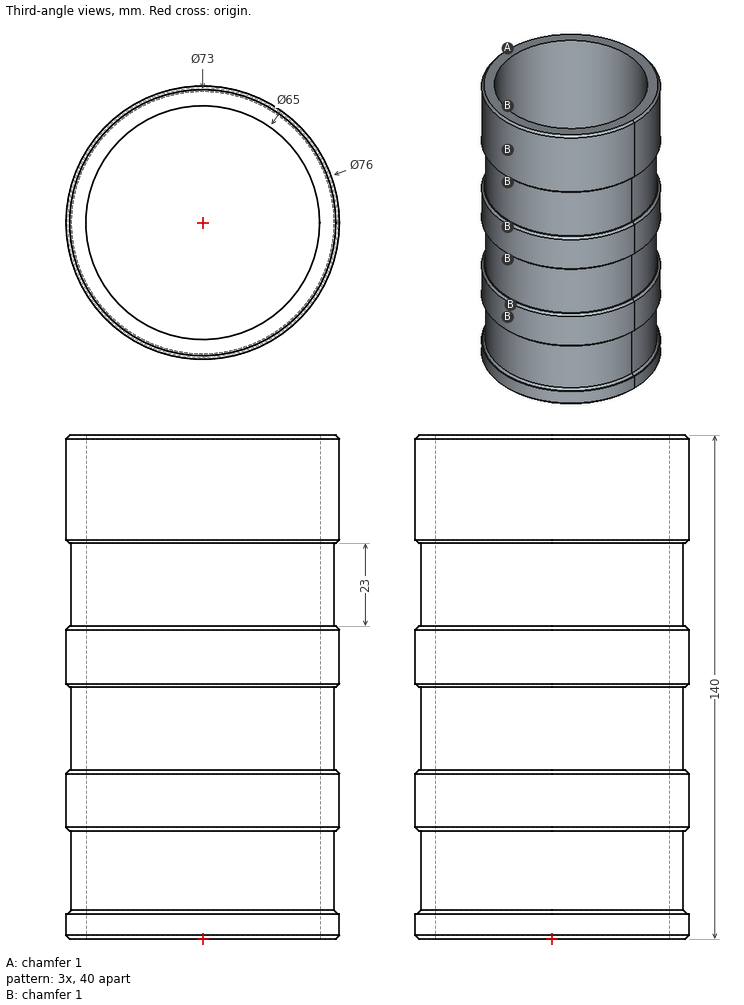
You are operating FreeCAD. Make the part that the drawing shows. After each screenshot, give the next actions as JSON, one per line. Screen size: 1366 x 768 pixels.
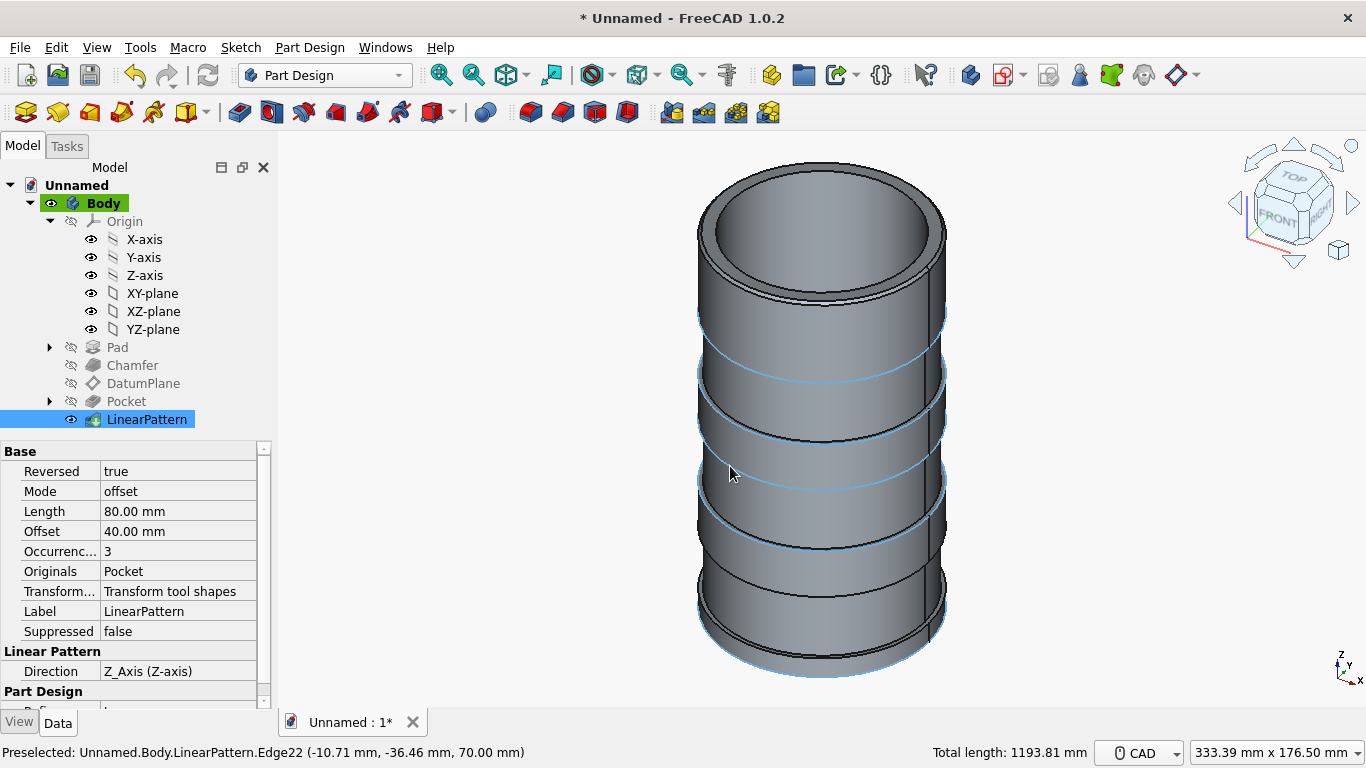
{"action": "left_click", "coordinate": [730, 573], "text": "ctrl"}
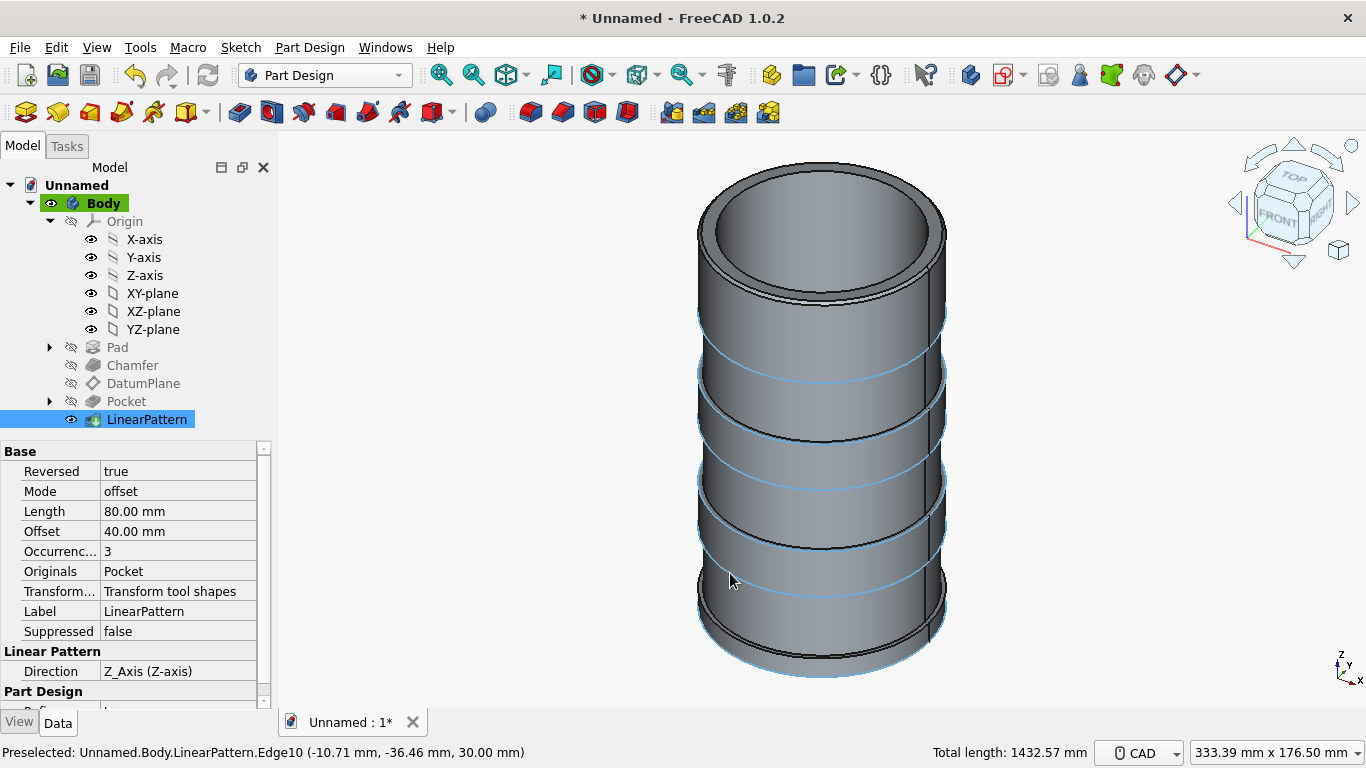
{"action": "key", "text": "0"}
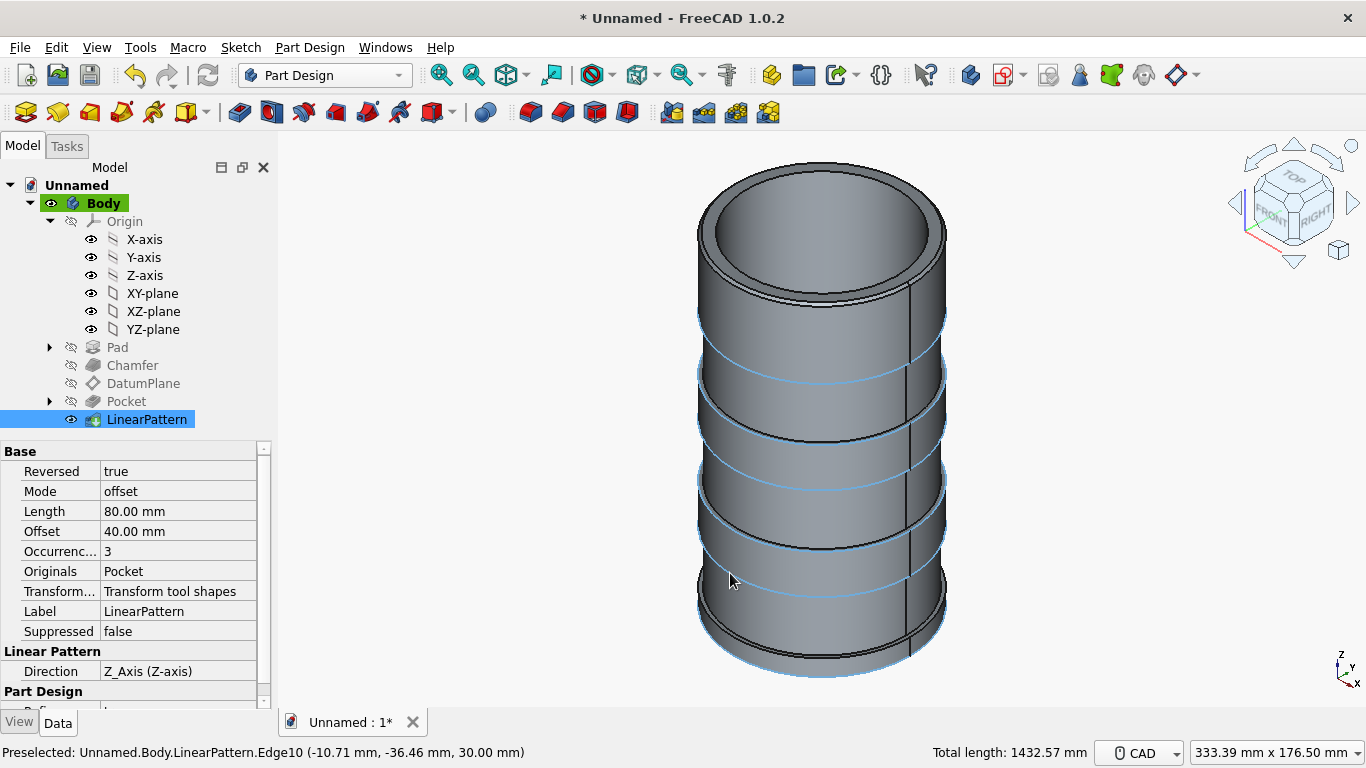
{"action": "left_click", "coordinate": [442, 76]}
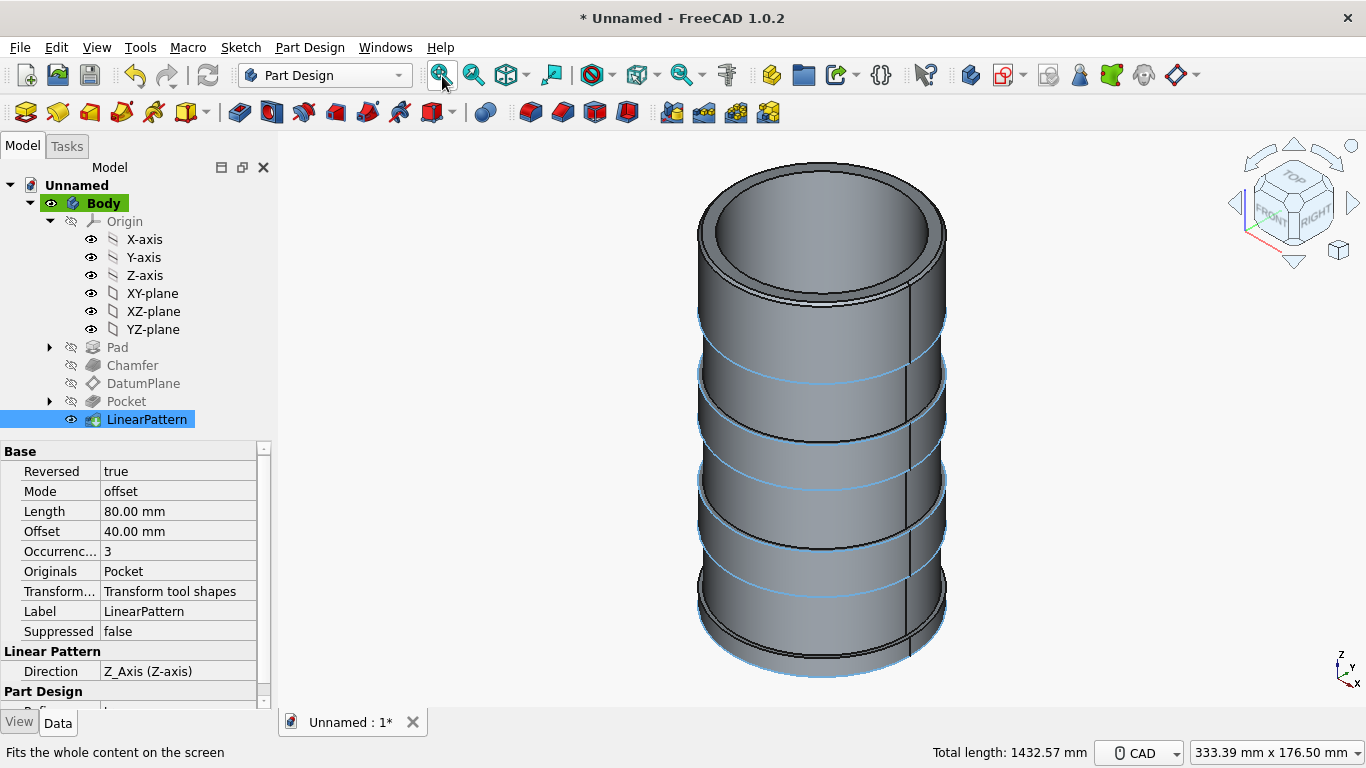
{"action": "key", "text": "2"}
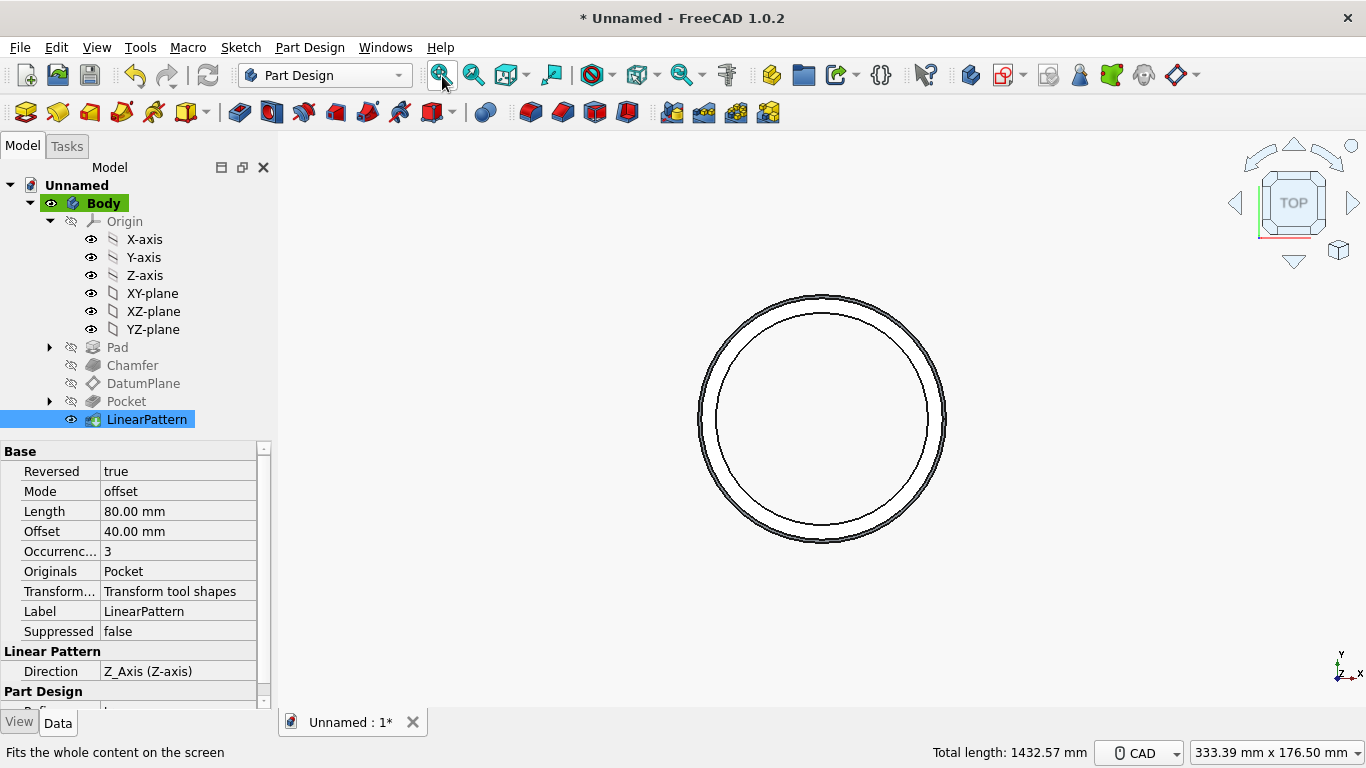
{"action": "key", "text": "v f"}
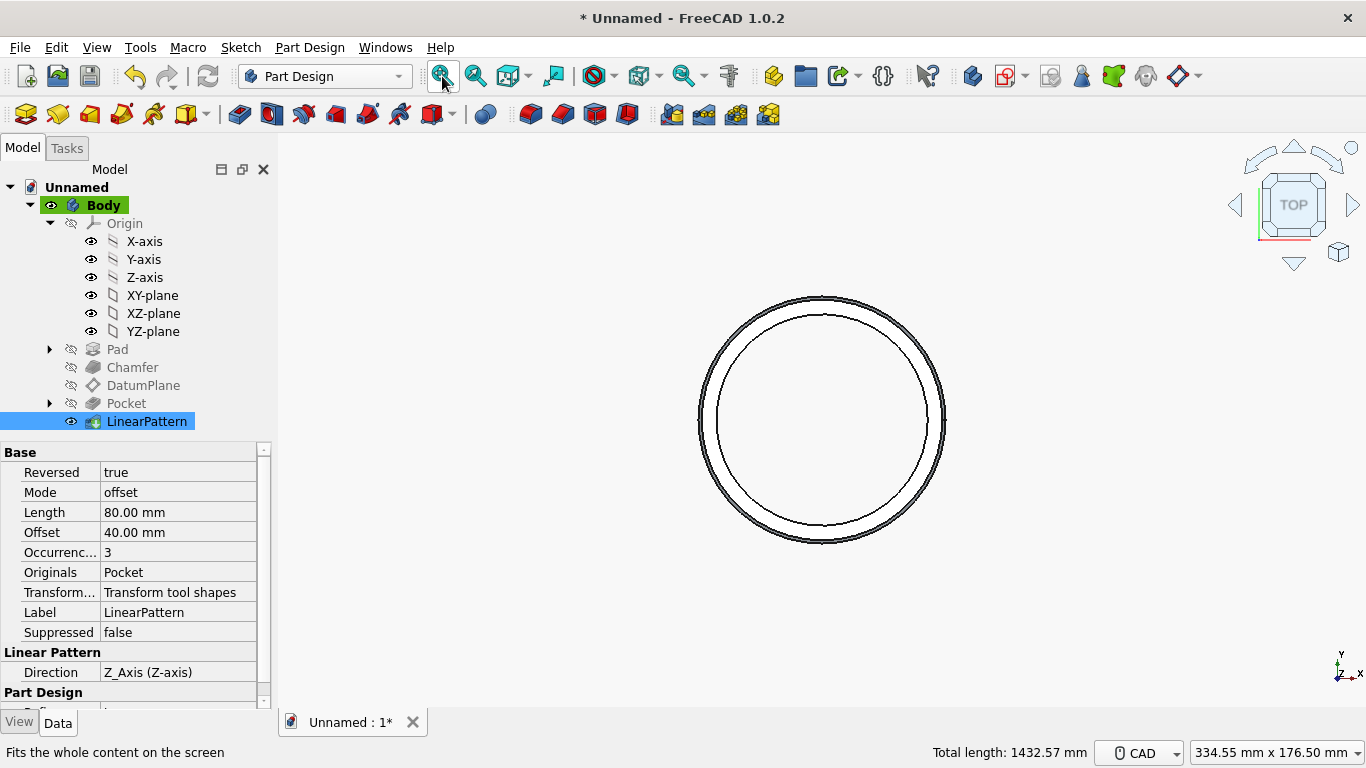
{"action": "key", "text": "1"}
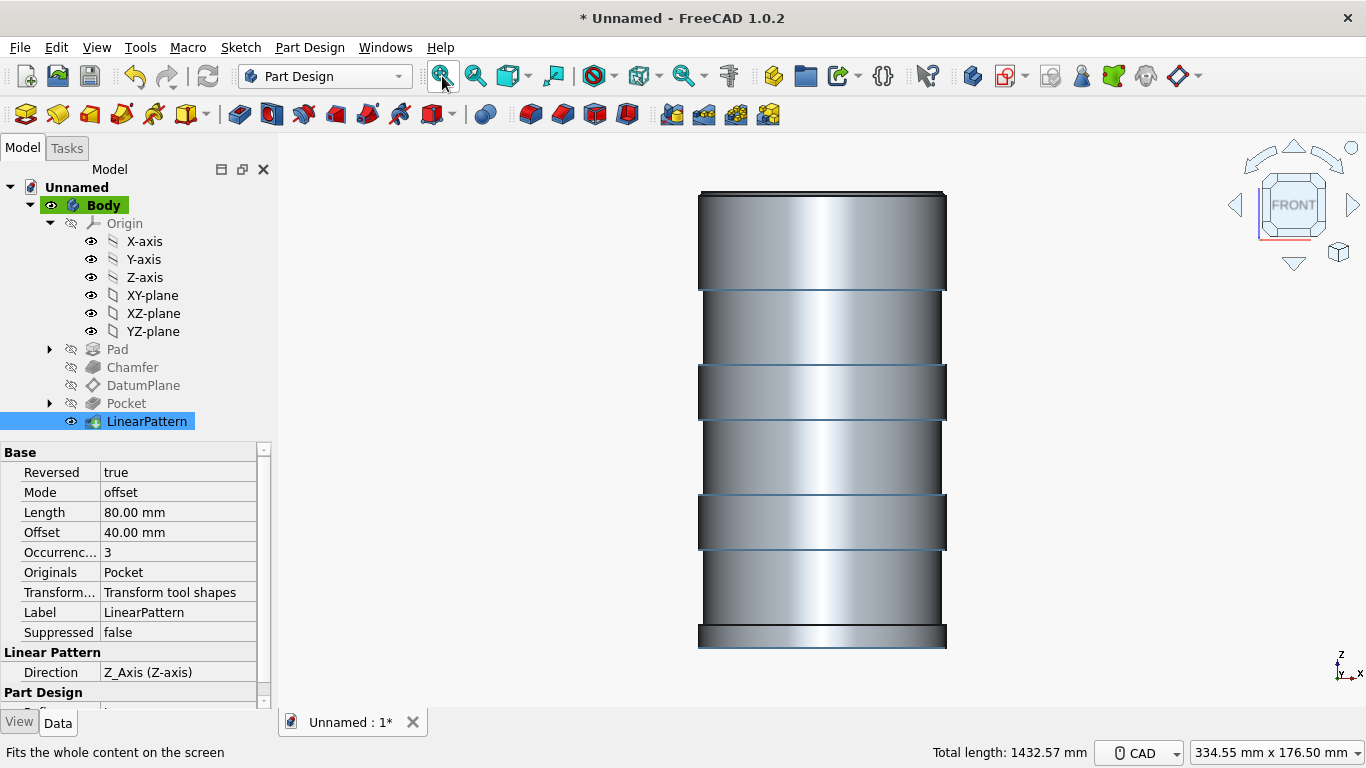
{"action": "key", "text": "3"}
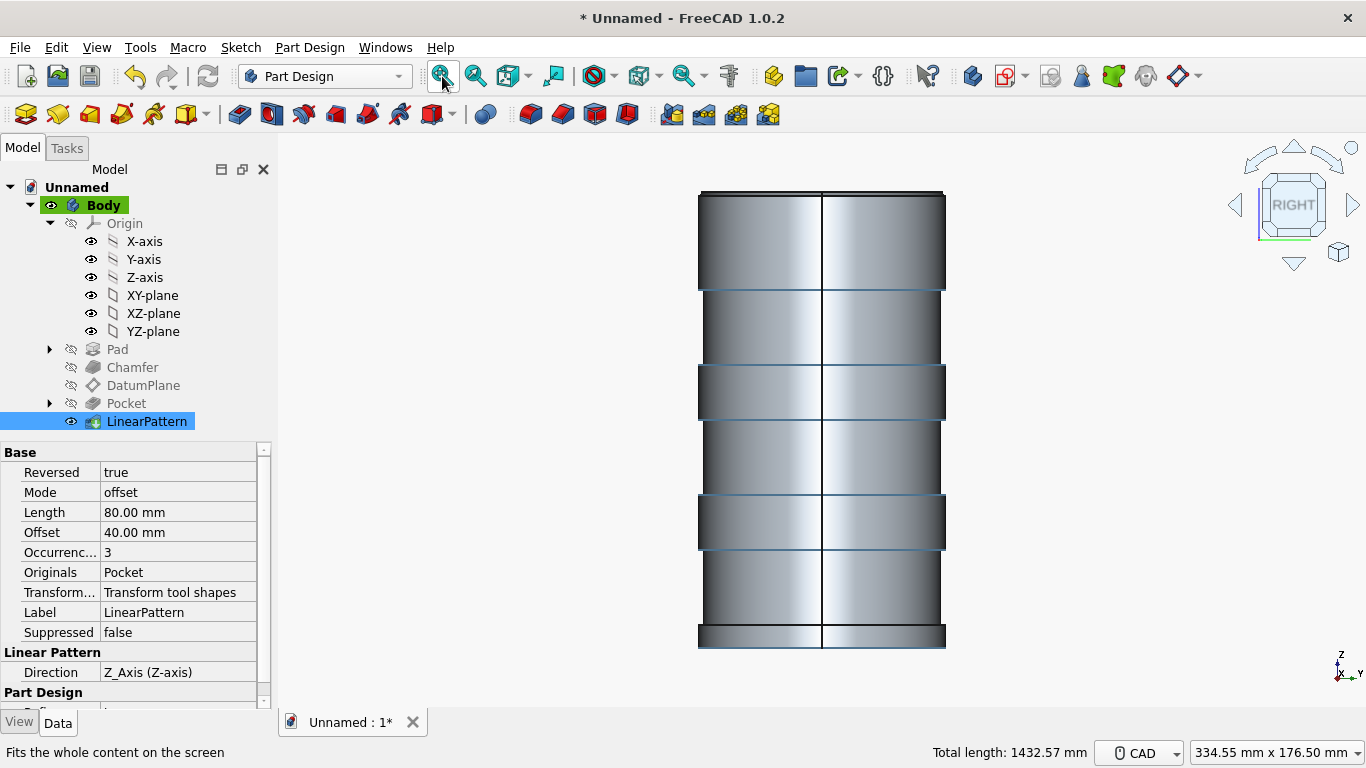
{"action": "key", "text": "5"}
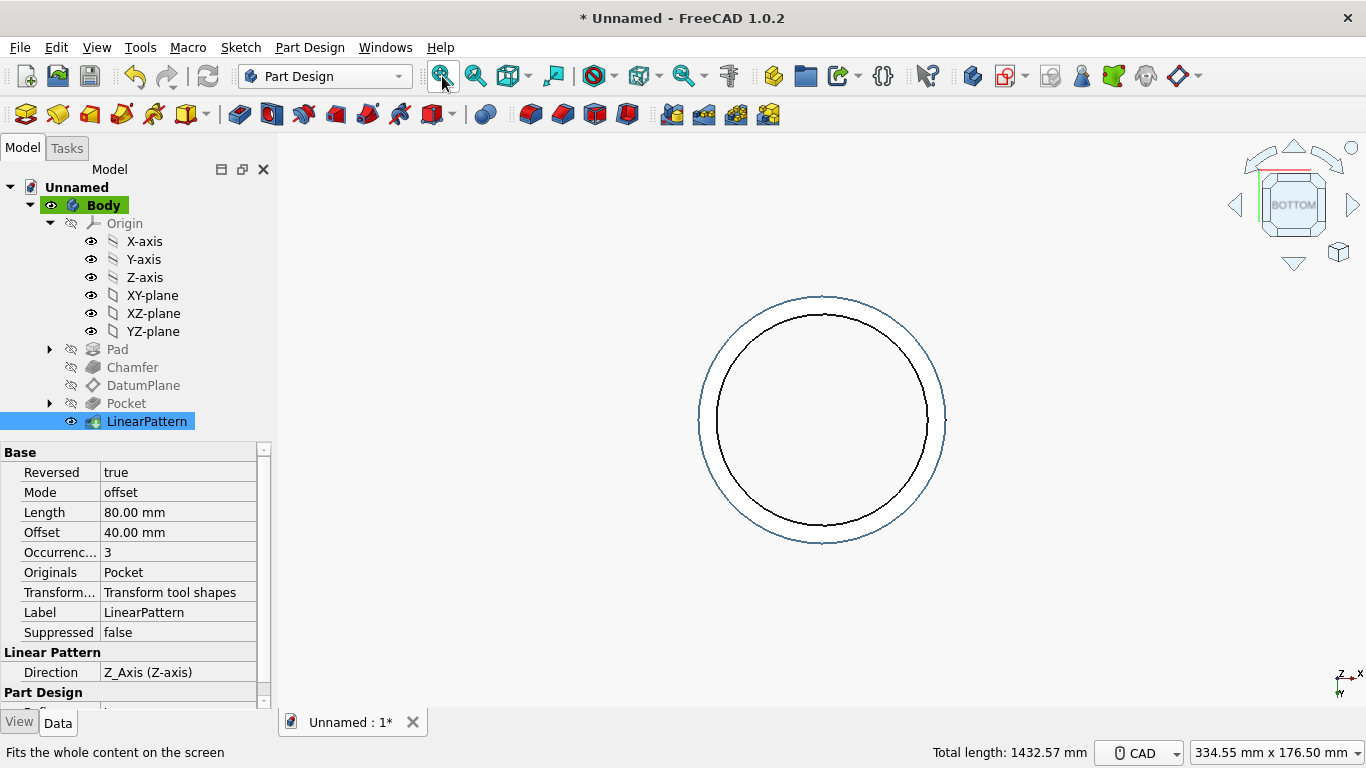
{"action": "key", "text": "v f"}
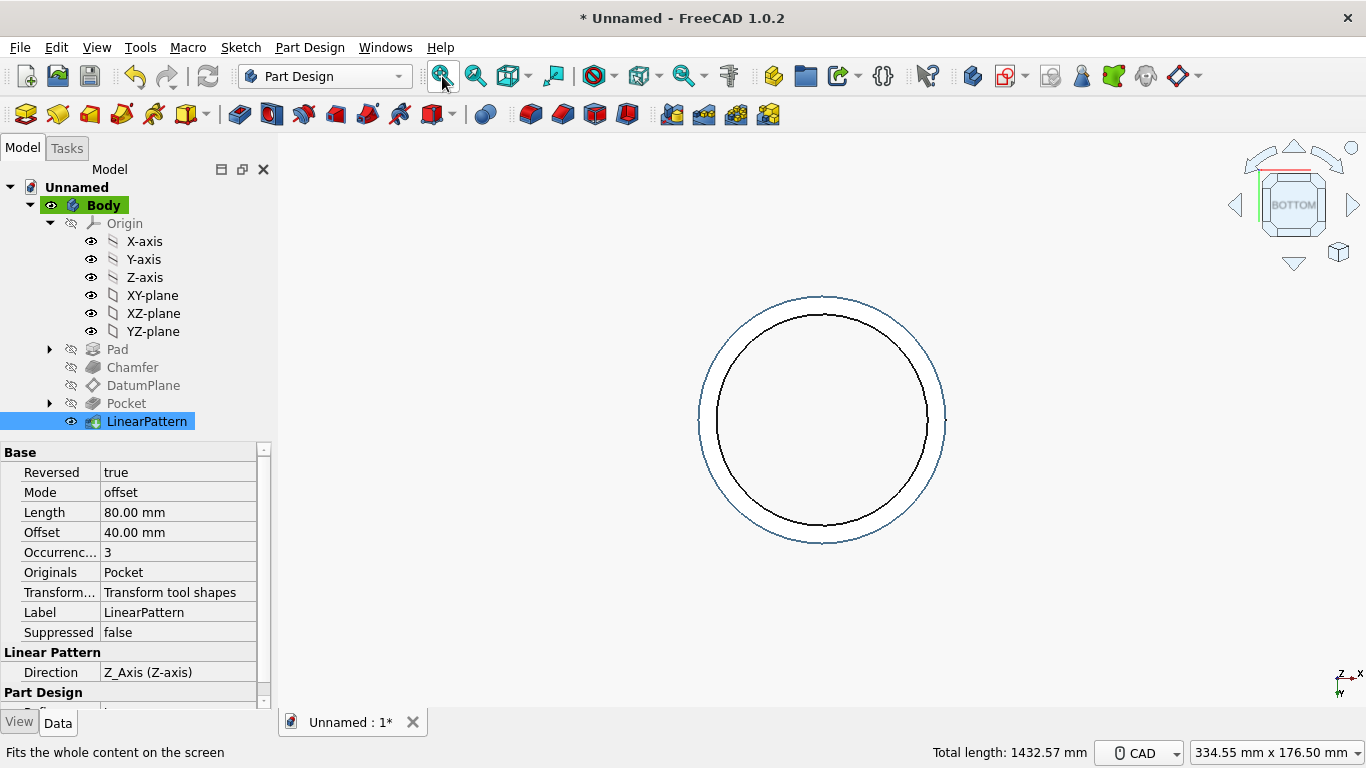
{"action": "key", "text": "4"}